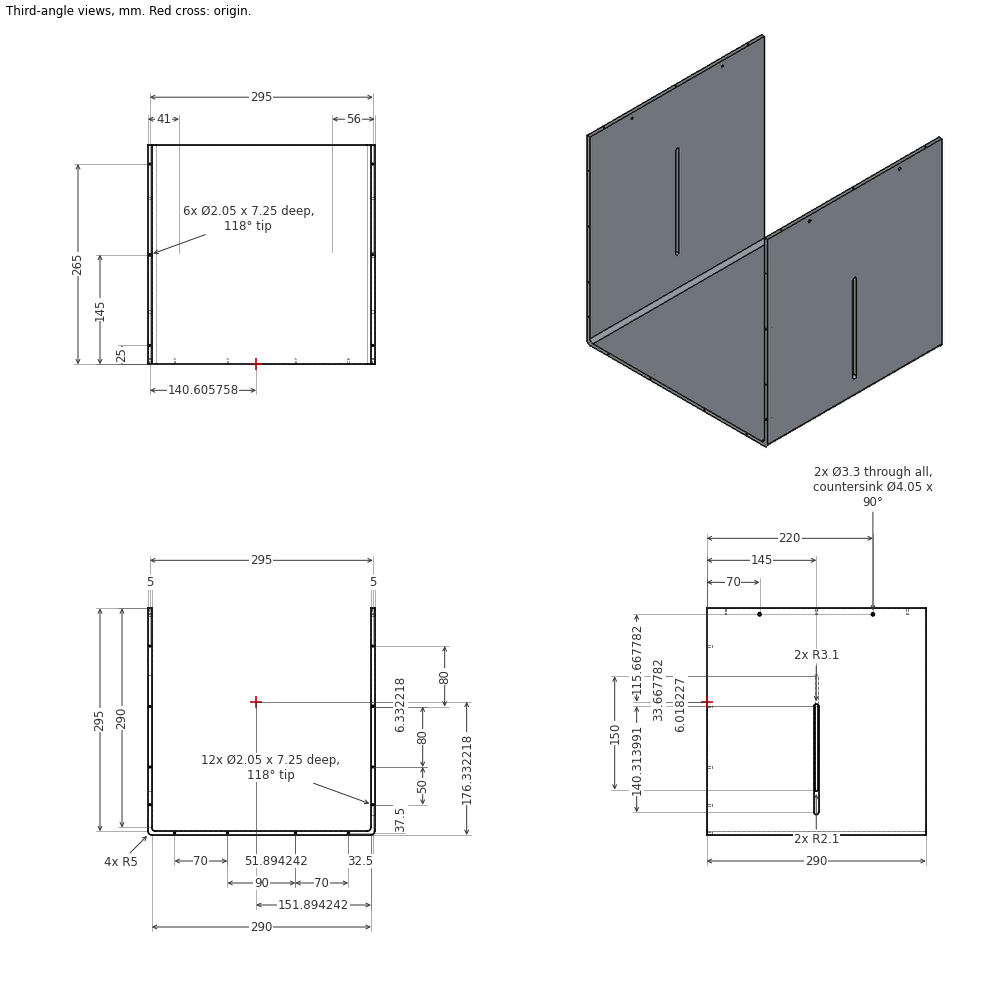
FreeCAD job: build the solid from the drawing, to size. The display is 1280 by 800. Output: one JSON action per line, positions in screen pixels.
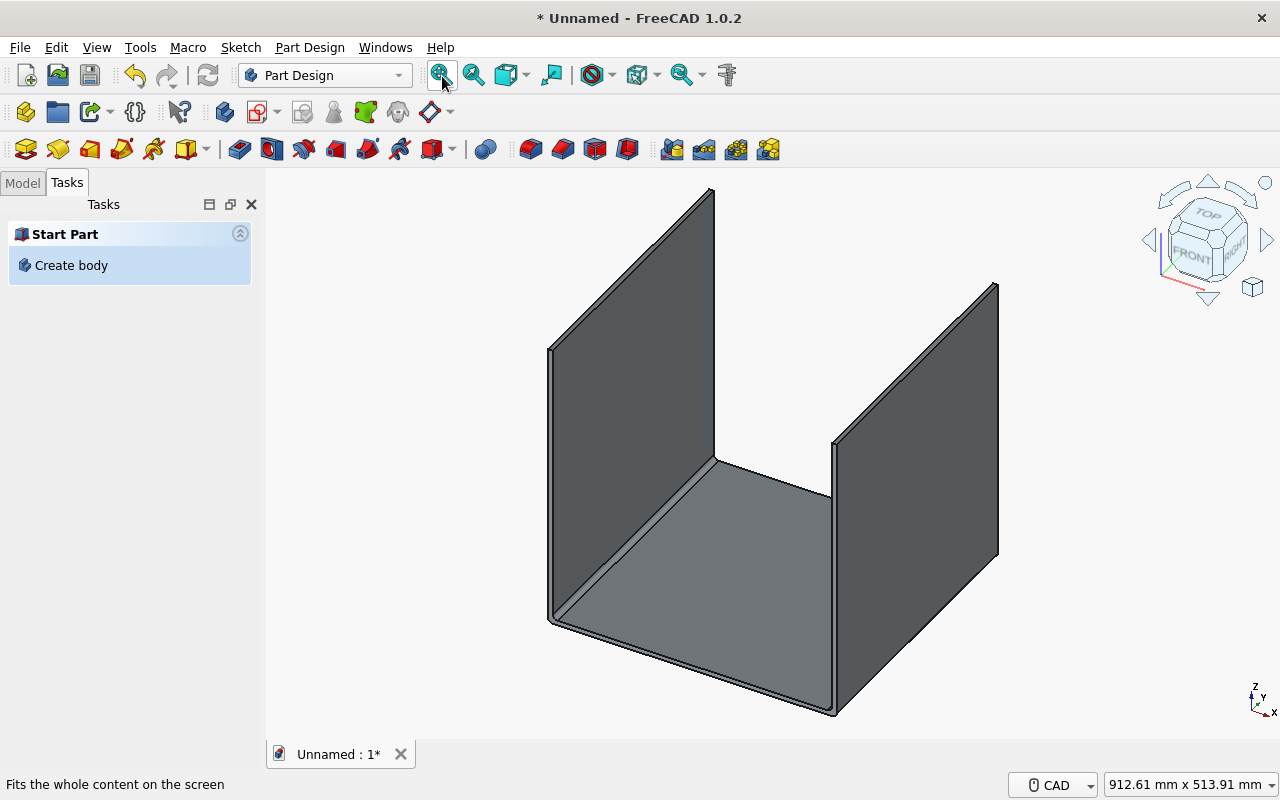
{"action": "scroll", "coordinate": [700, 200], "scroll_direction": "up", "scroll_amount": 8}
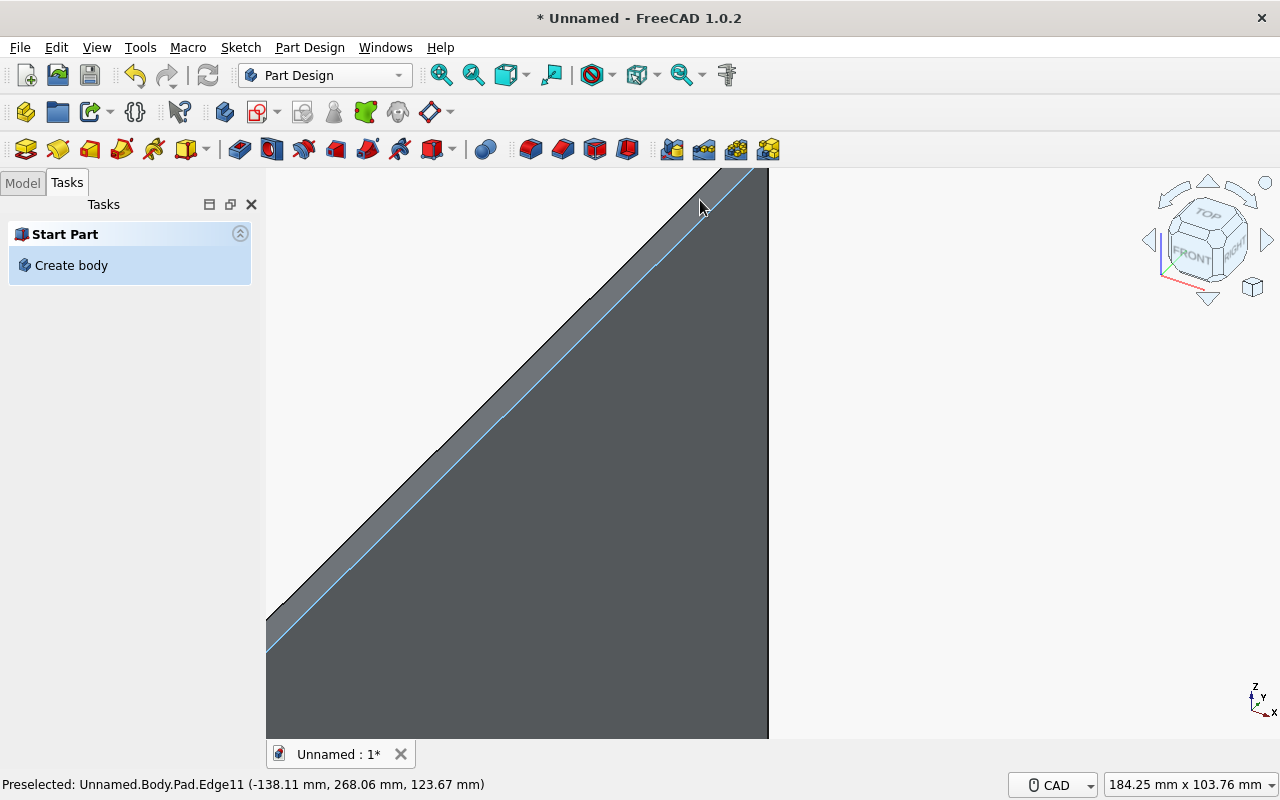
{"action": "left_click", "coordinate": [699, 206]}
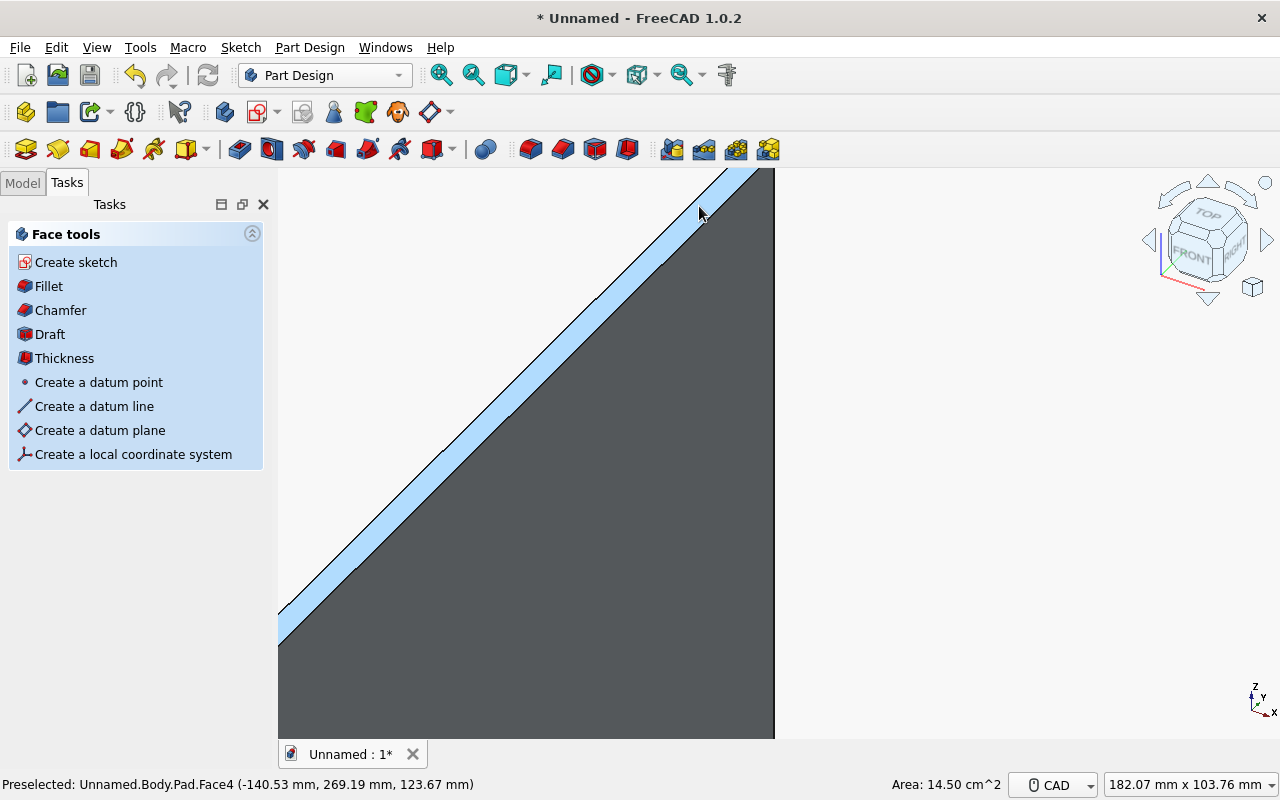
{"action": "left_click", "coordinate": [258, 112]}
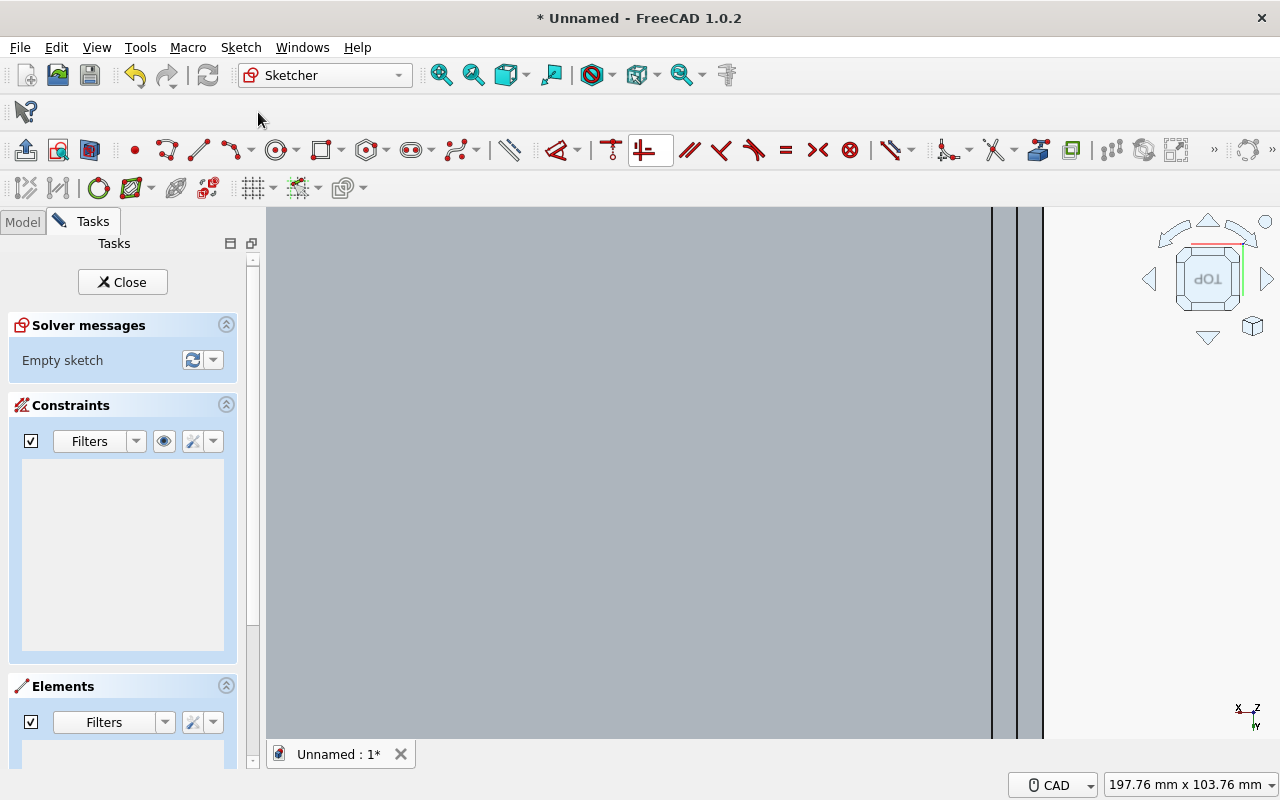
{"action": "scroll", "coordinate": [845, 601], "scroll_direction": "down", "scroll_amount": 7}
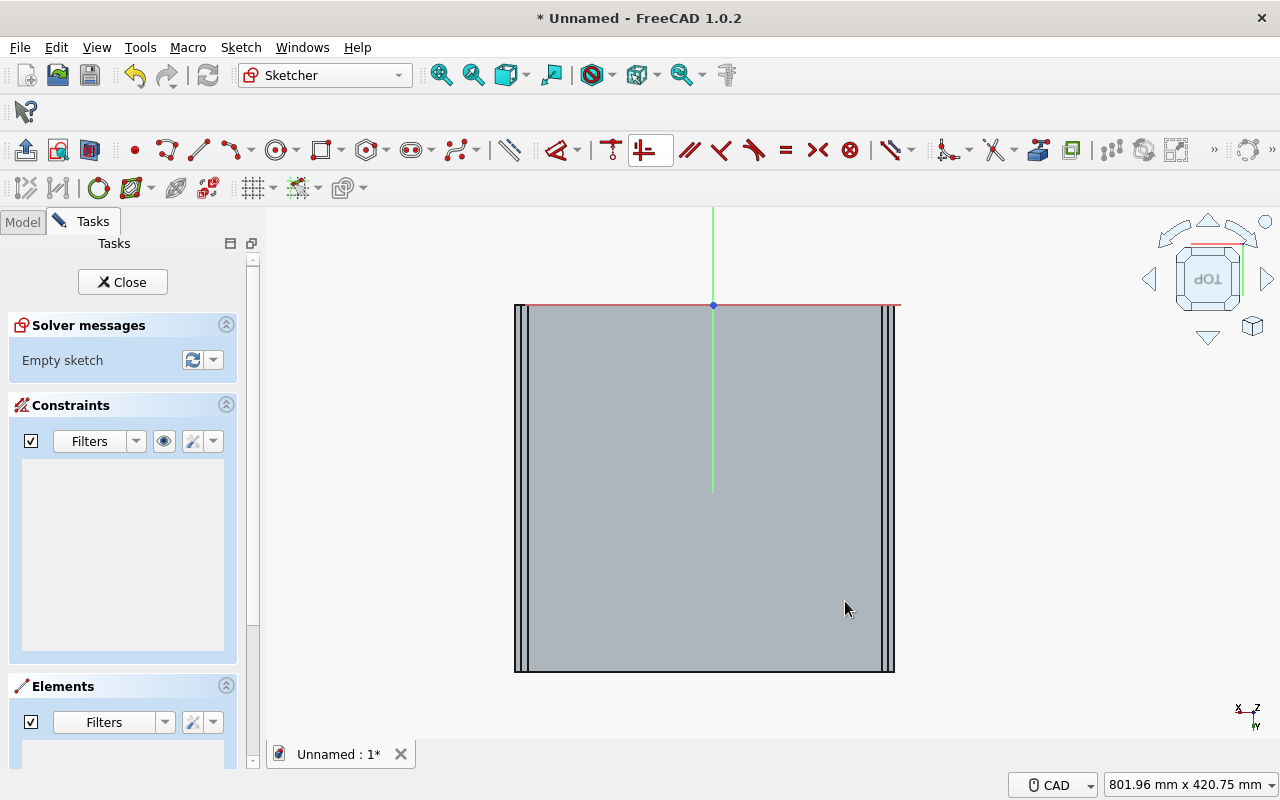
{"action": "left_click", "coordinate": [276, 150]}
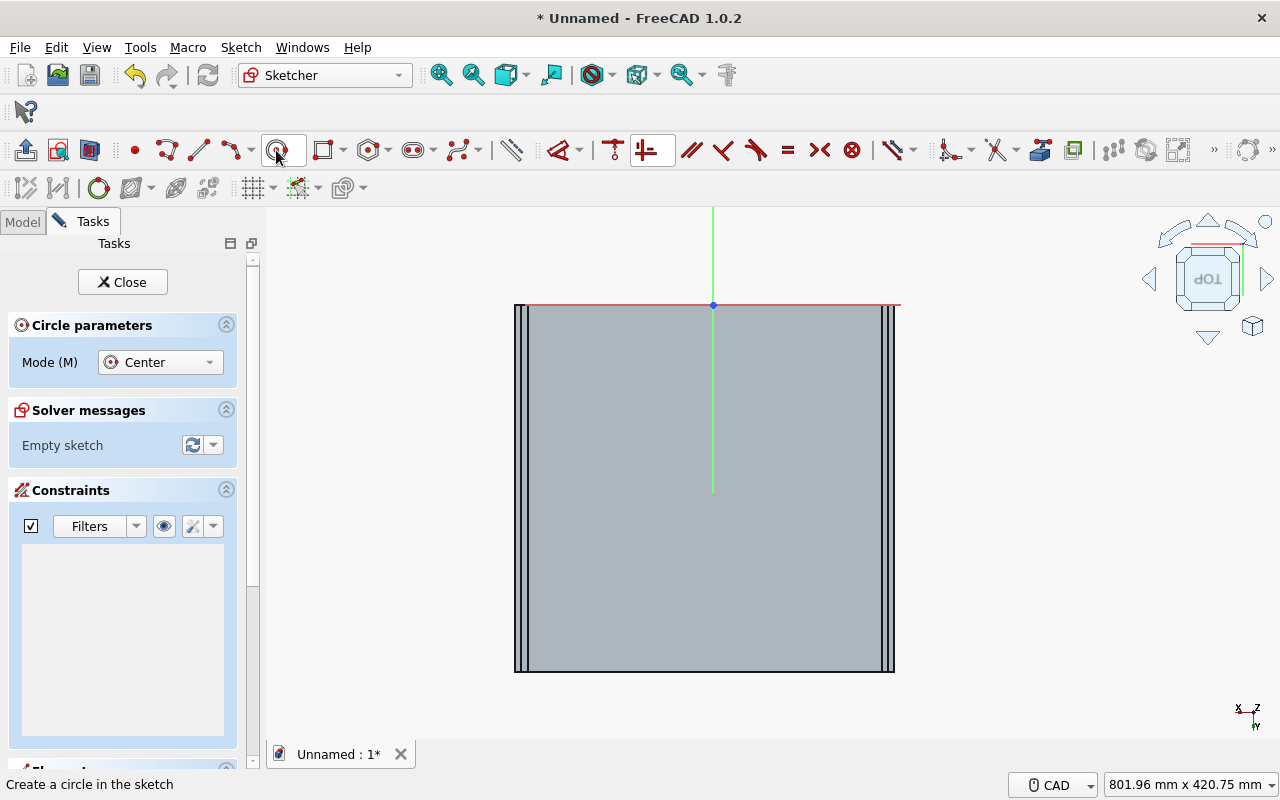
{"action": "scroll", "coordinate": [891, 489], "scroll_direction": "up", "scroll_amount": 15}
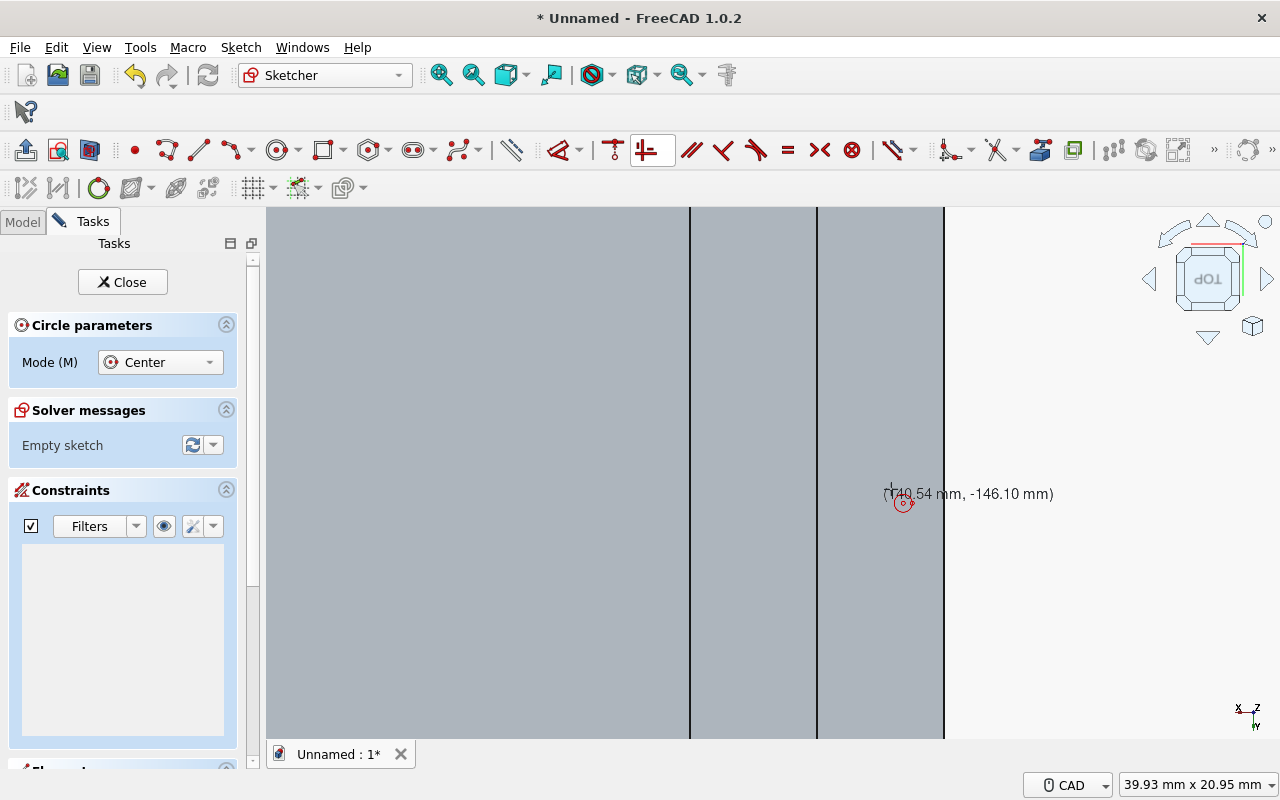
{"action": "scroll", "coordinate": [892, 489], "scroll_direction": "down", "scroll_amount": 15}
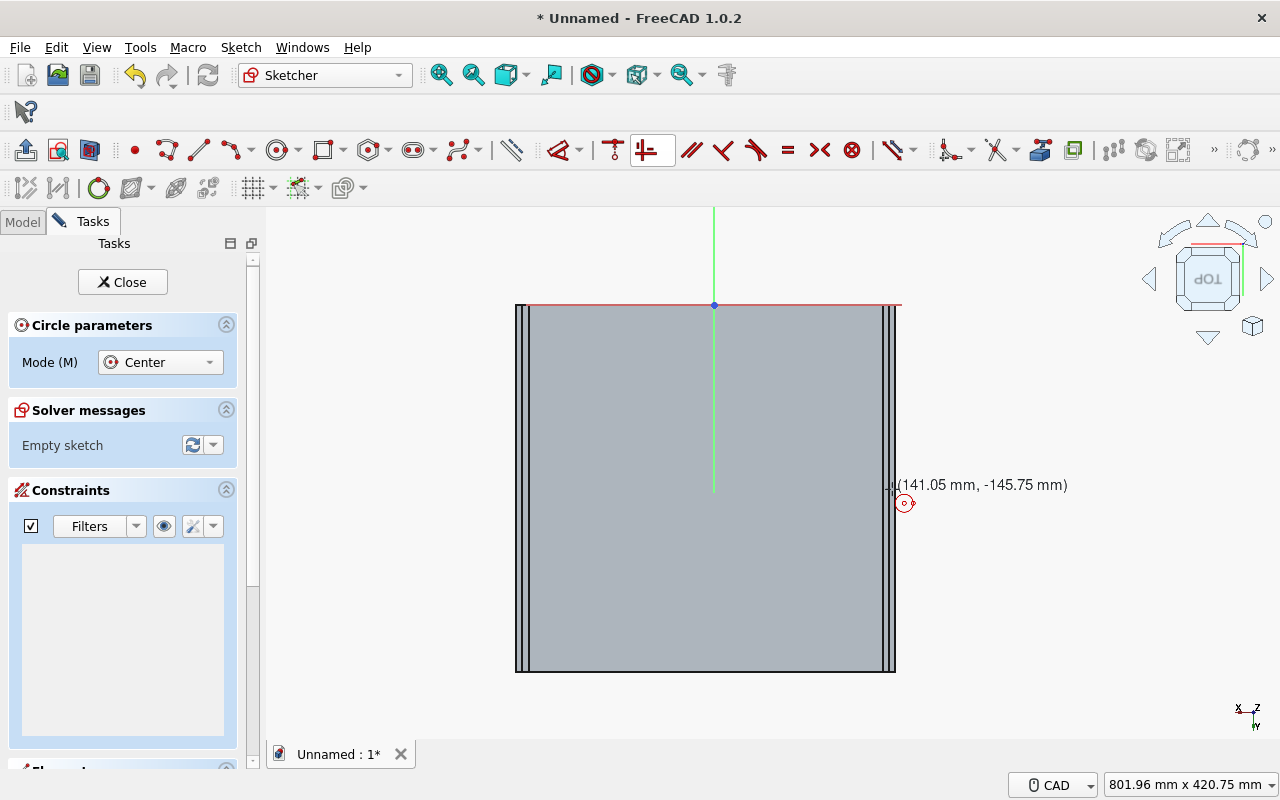
{"action": "left_click", "coordinate": [892, 489]}
{"action": "mouse_move", "coordinate": [893, 488]}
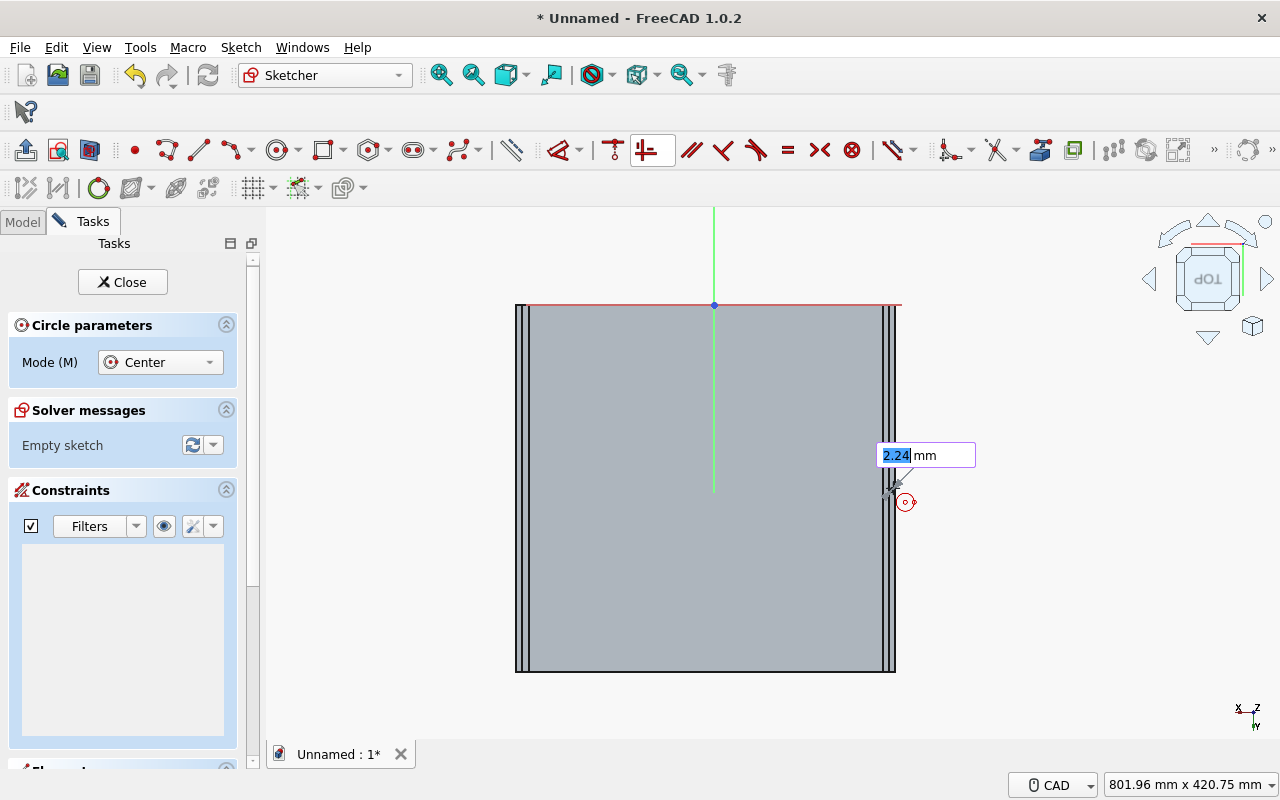
{"action": "type", "text": "2.05"}
{"action": "key", "text": "Return"}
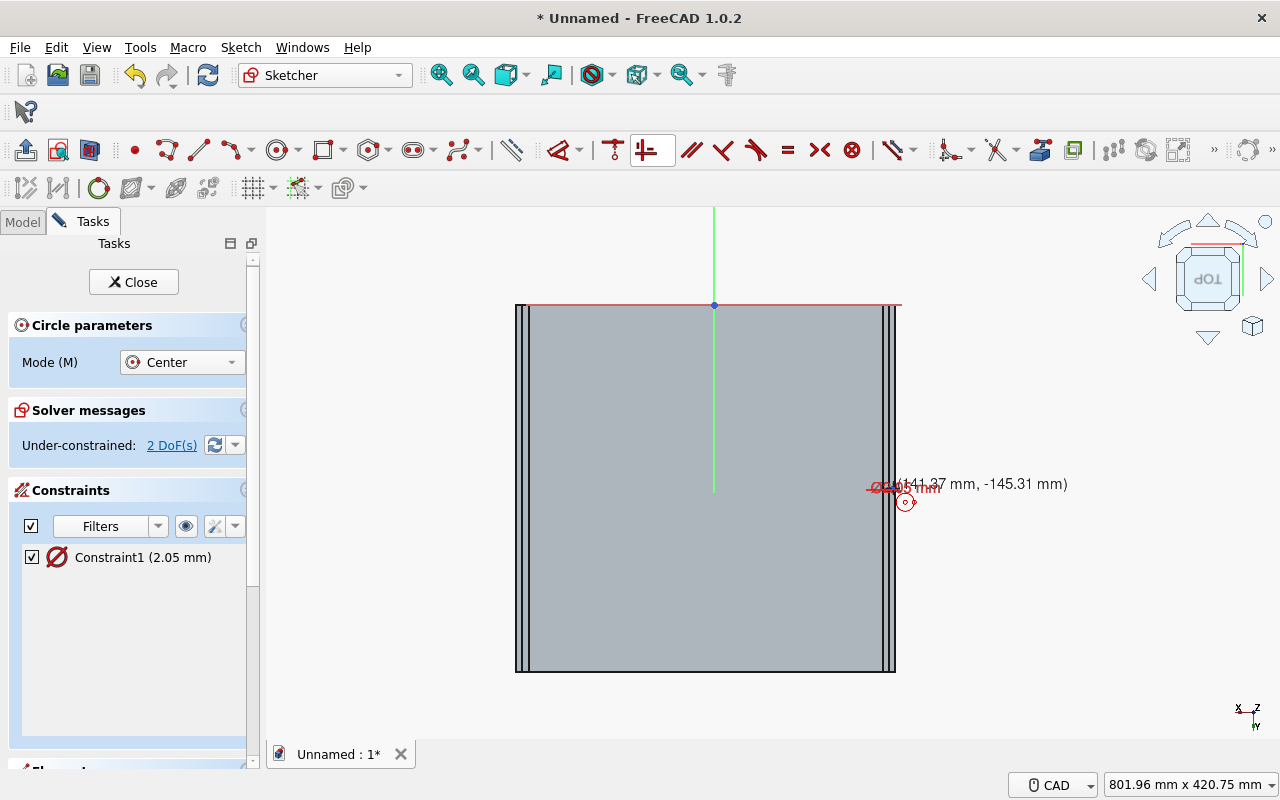
{"action": "scroll", "coordinate": [892, 640], "scroll_direction": "up", "scroll_amount": 15}